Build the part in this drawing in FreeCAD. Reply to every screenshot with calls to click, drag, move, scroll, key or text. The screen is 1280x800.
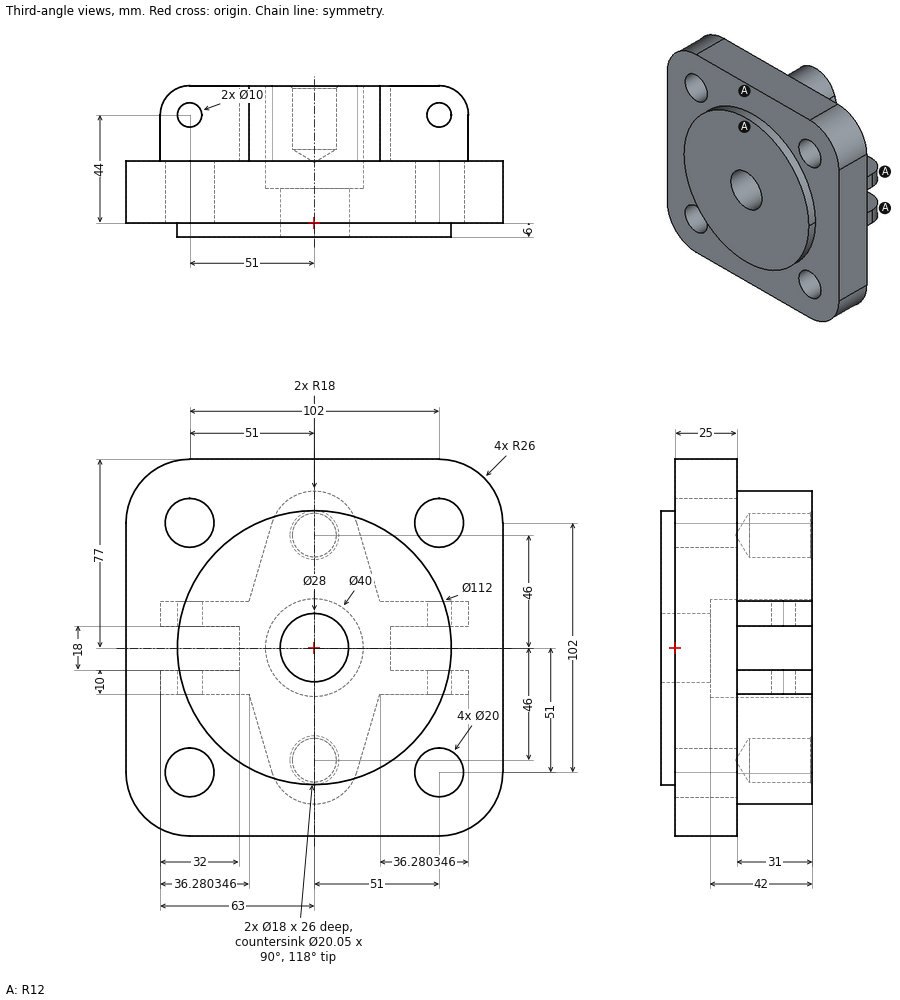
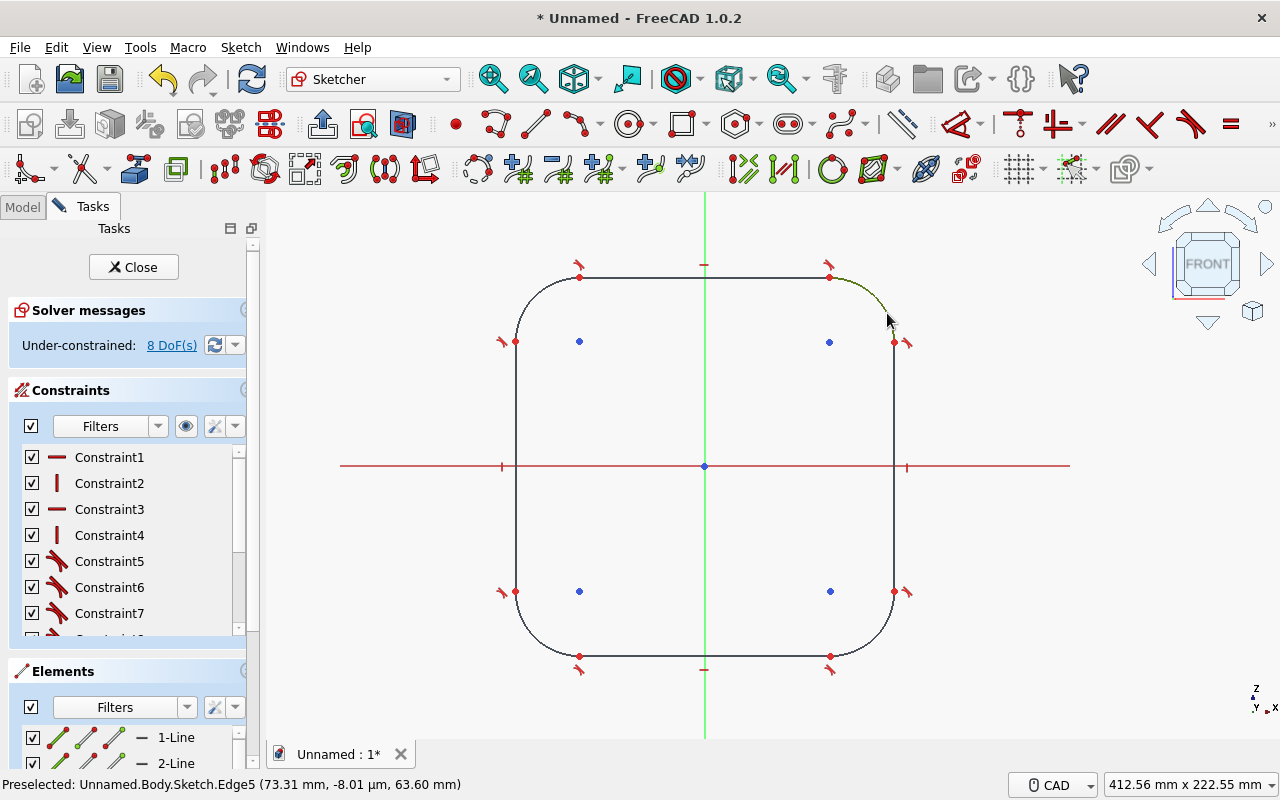
click(859, 649)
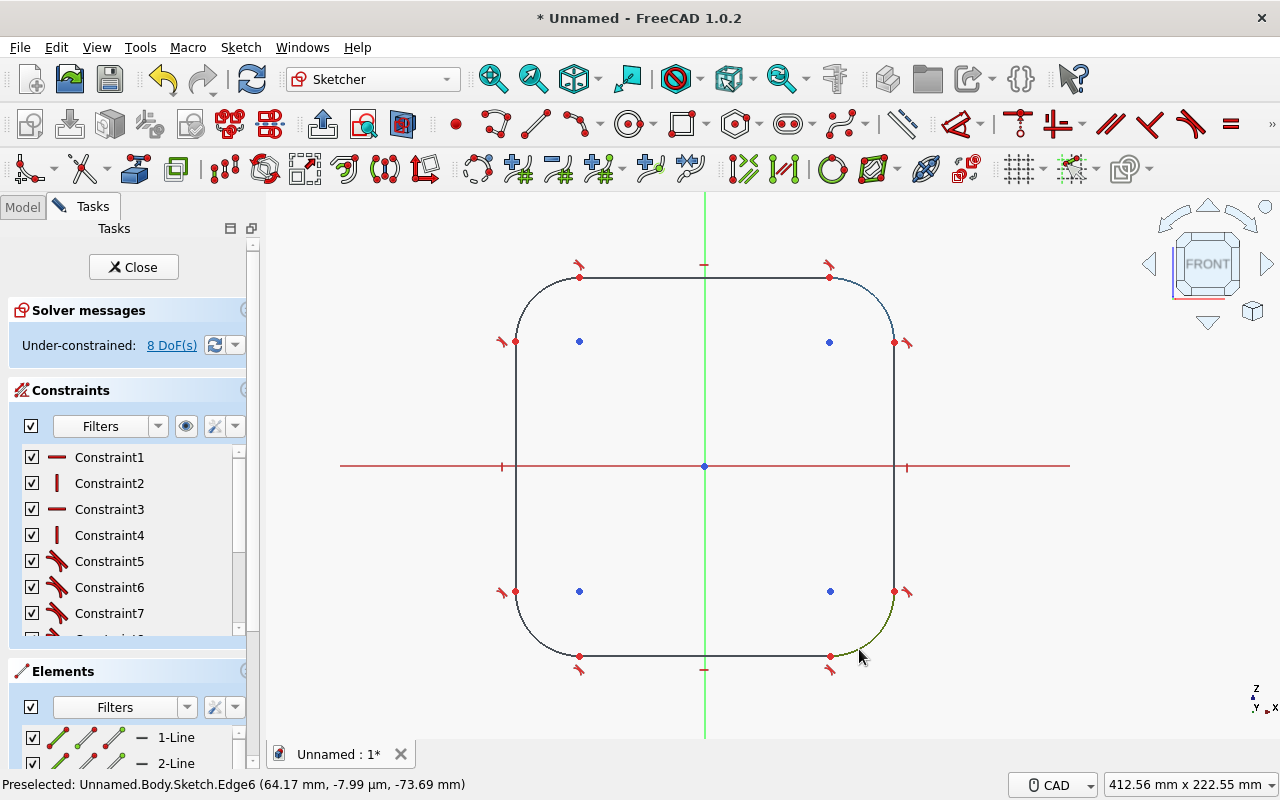
click(523, 621)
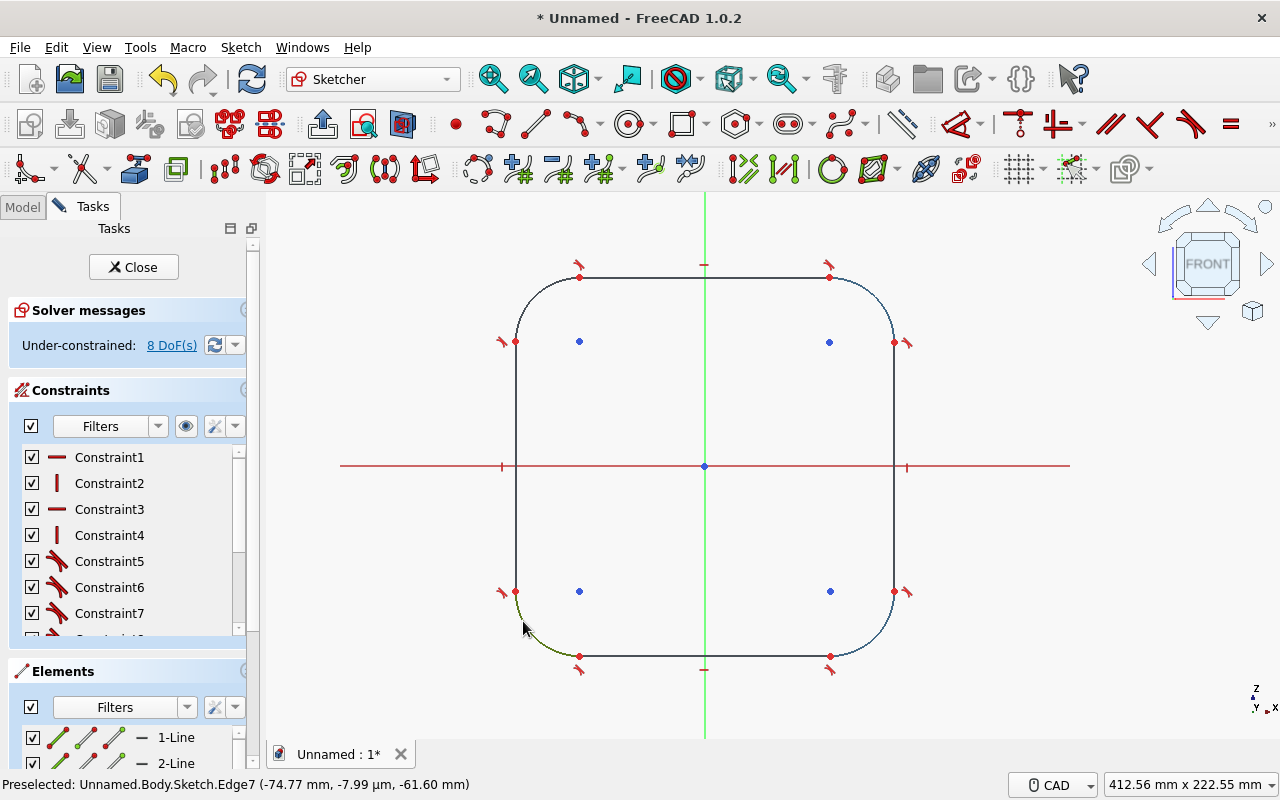
click(551, 285)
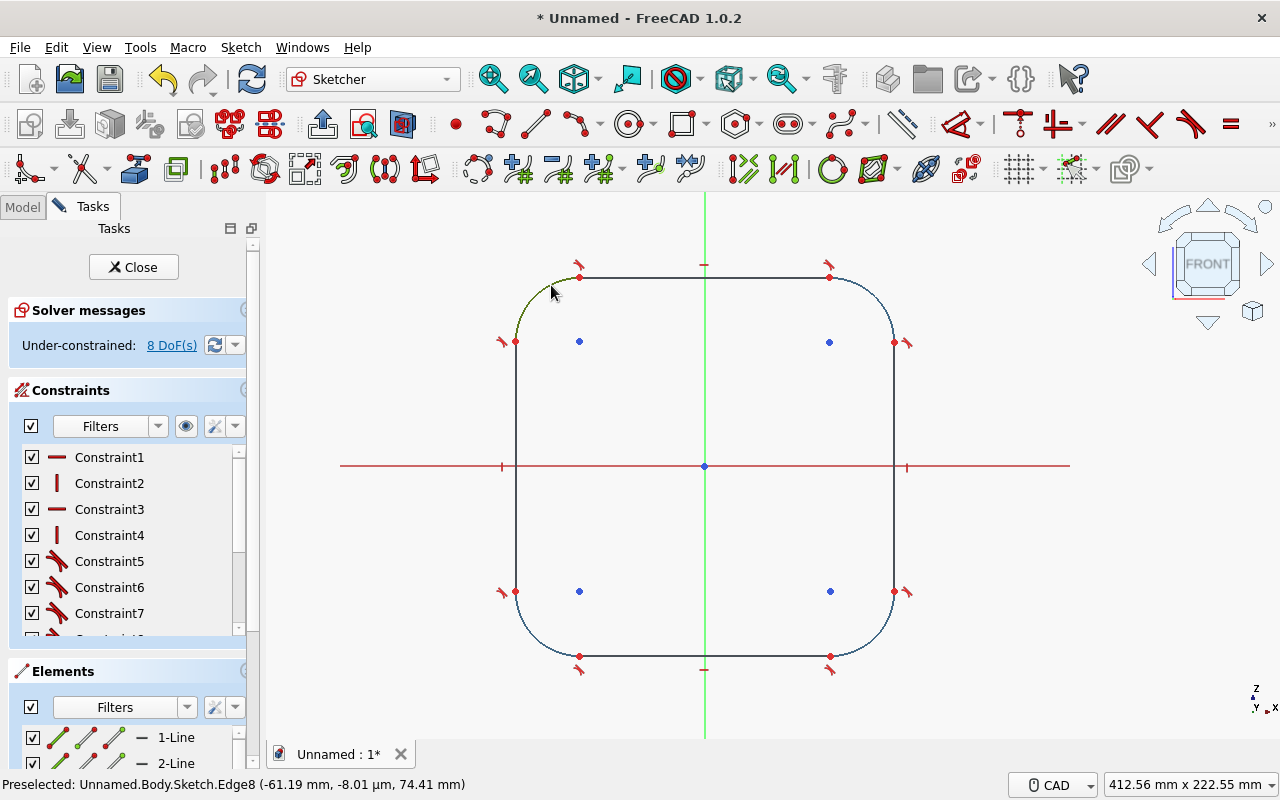
key(e)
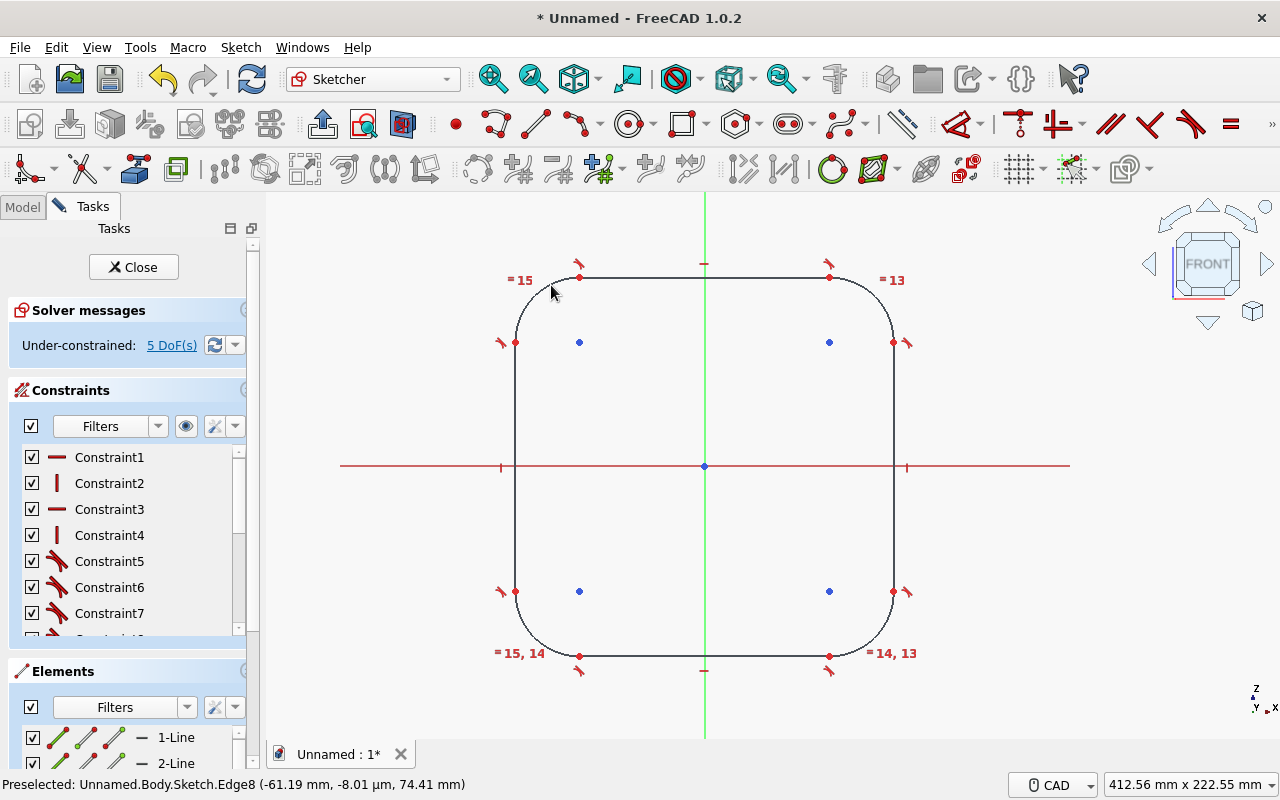
key(d)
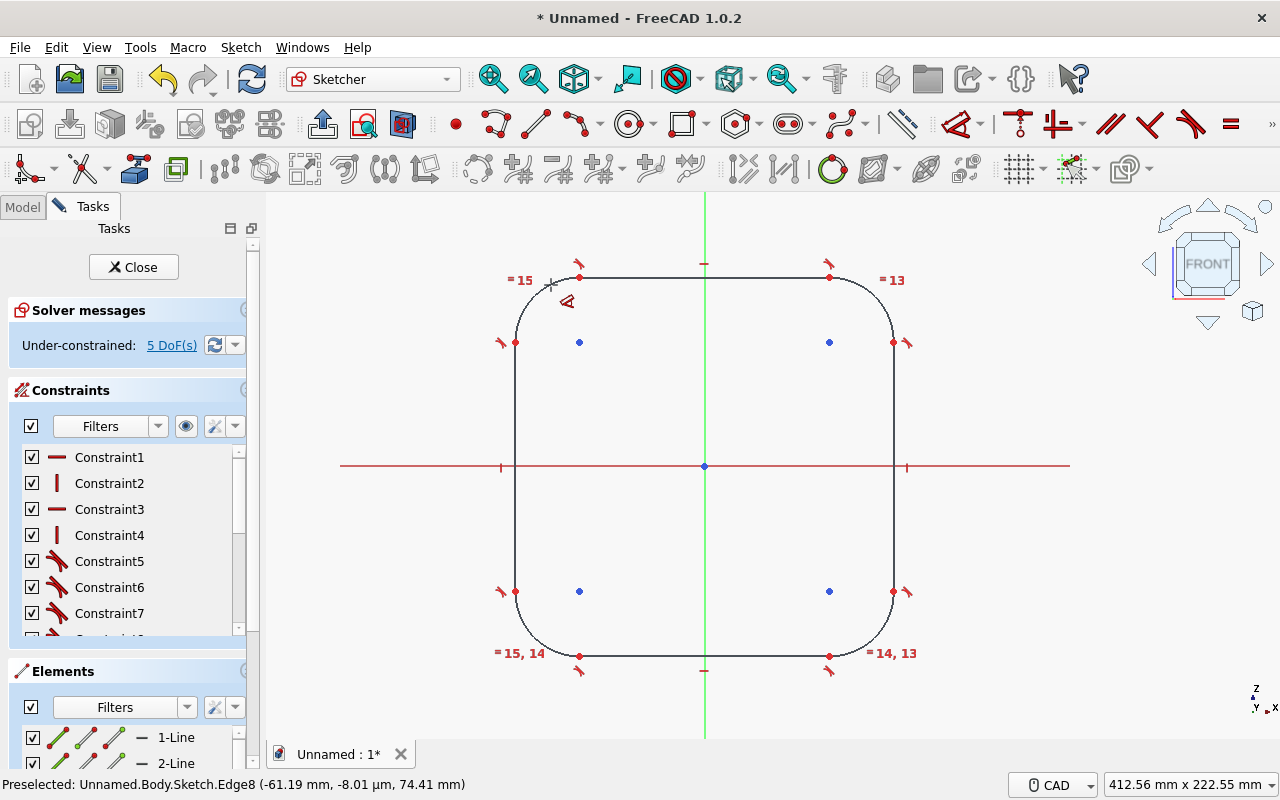
click(887, 313)
click(916, 299)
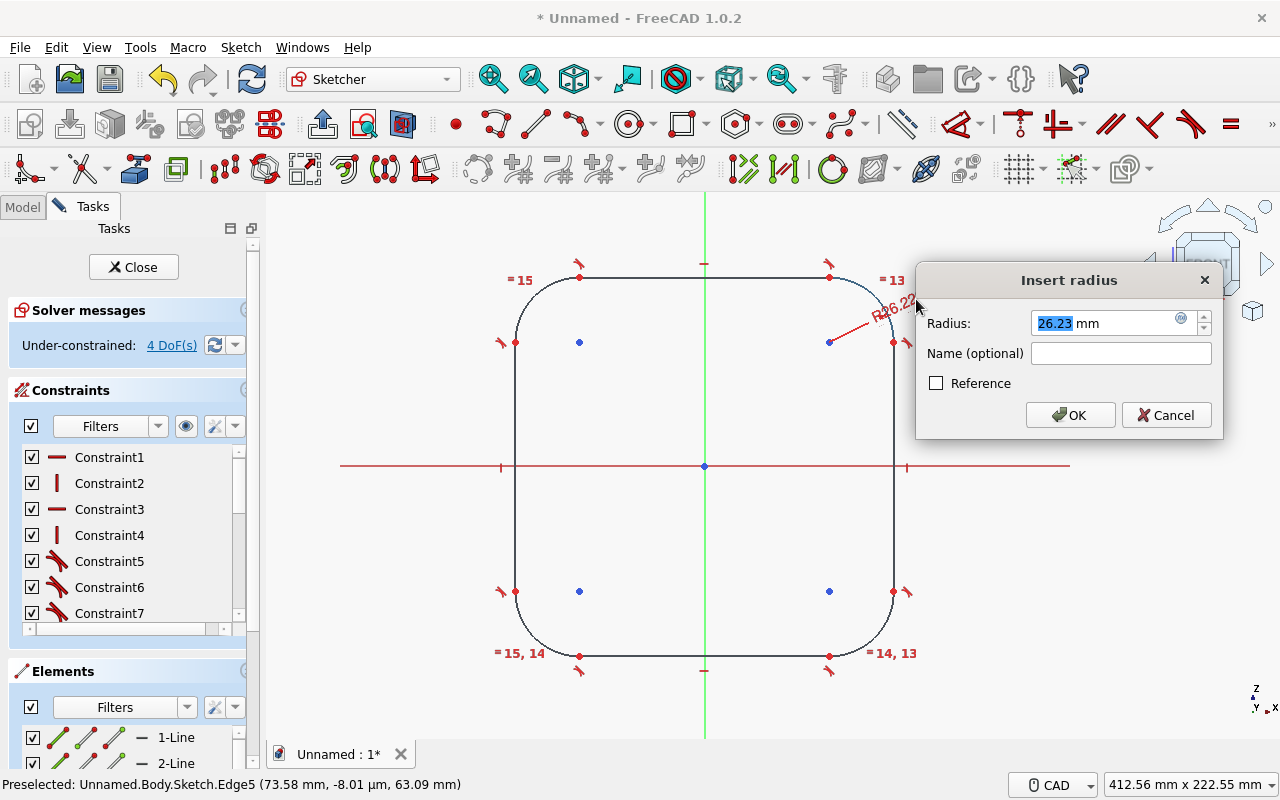
text(26)
key(Return)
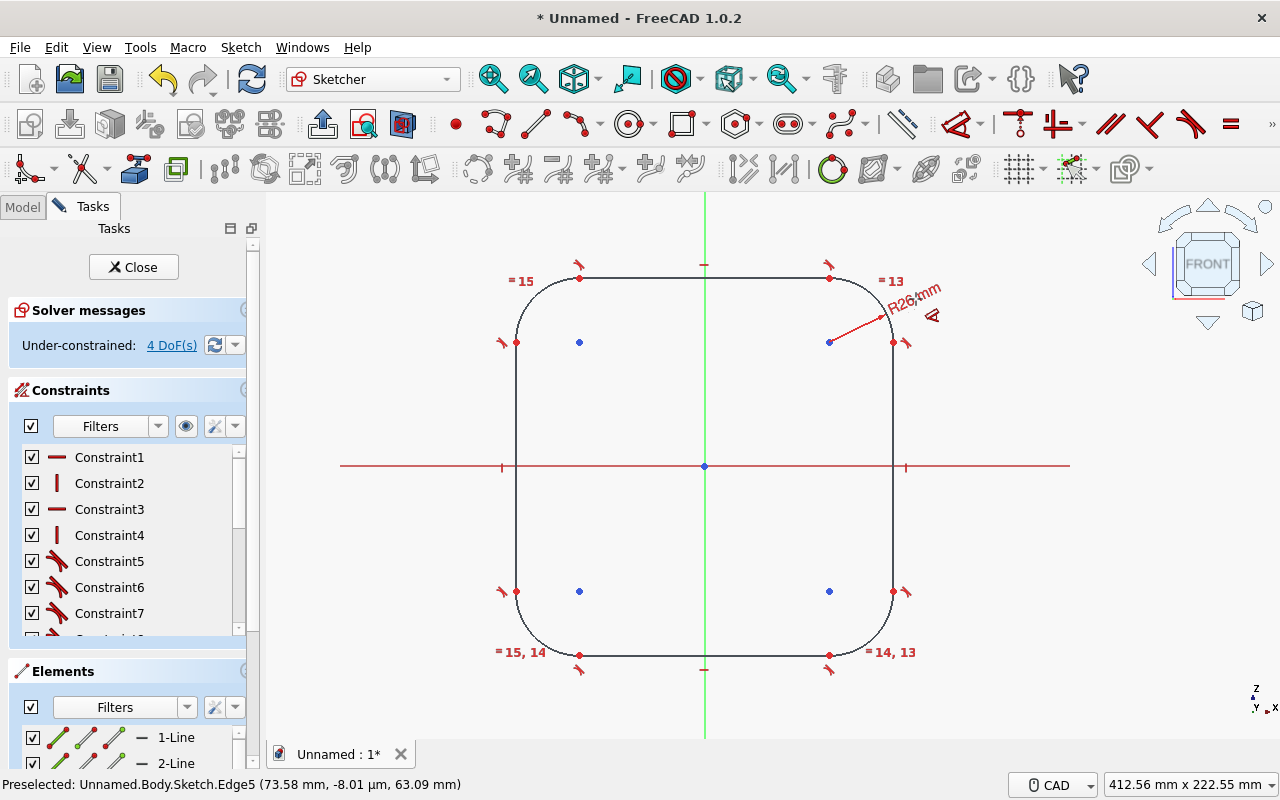
click(655, 278)
click(647, 244)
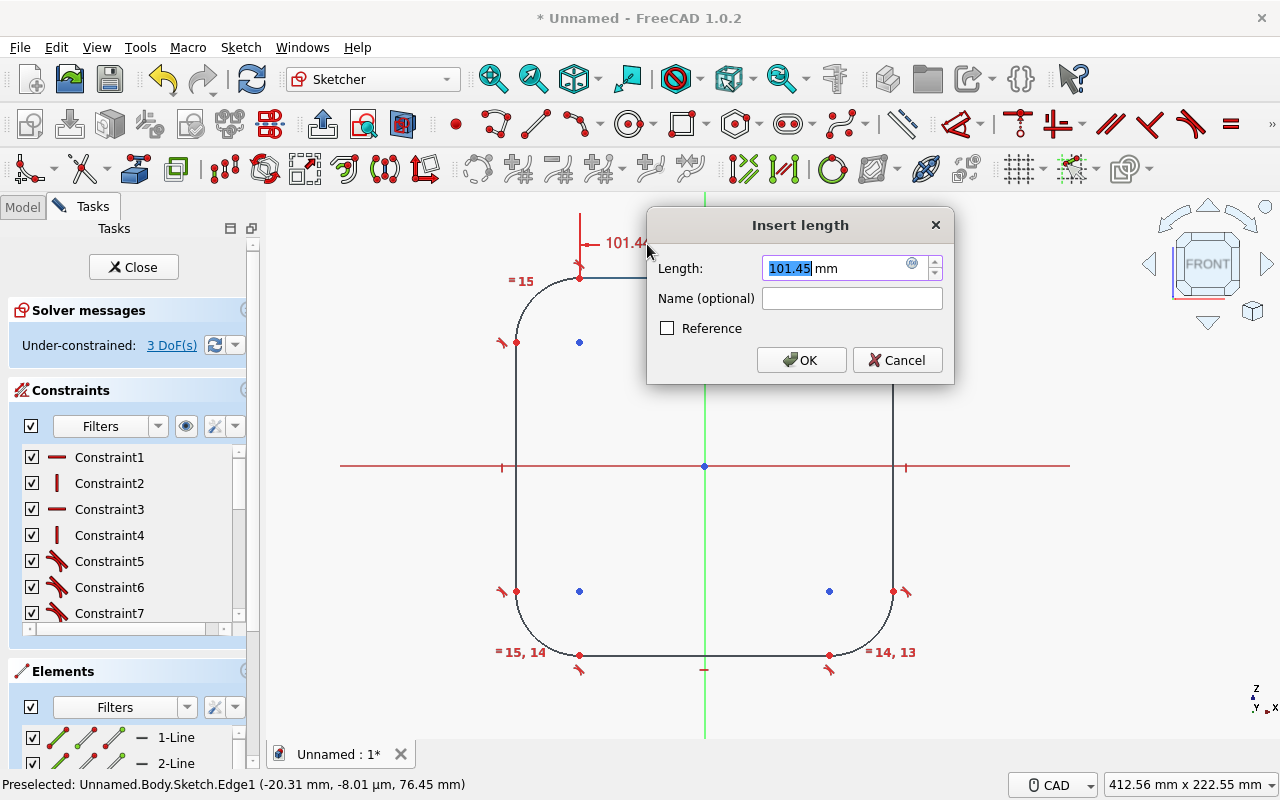
text(102)
key(Return)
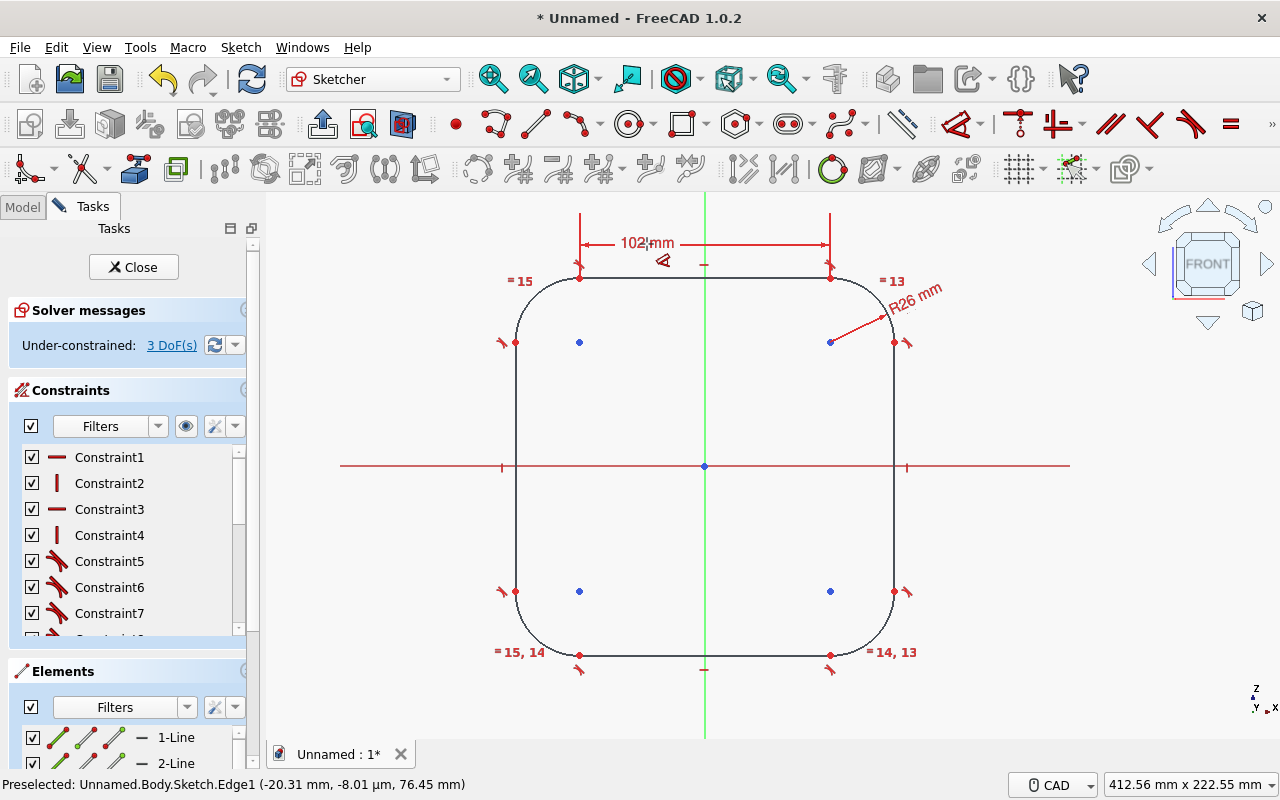
click(894, 417)
click(928, 410)